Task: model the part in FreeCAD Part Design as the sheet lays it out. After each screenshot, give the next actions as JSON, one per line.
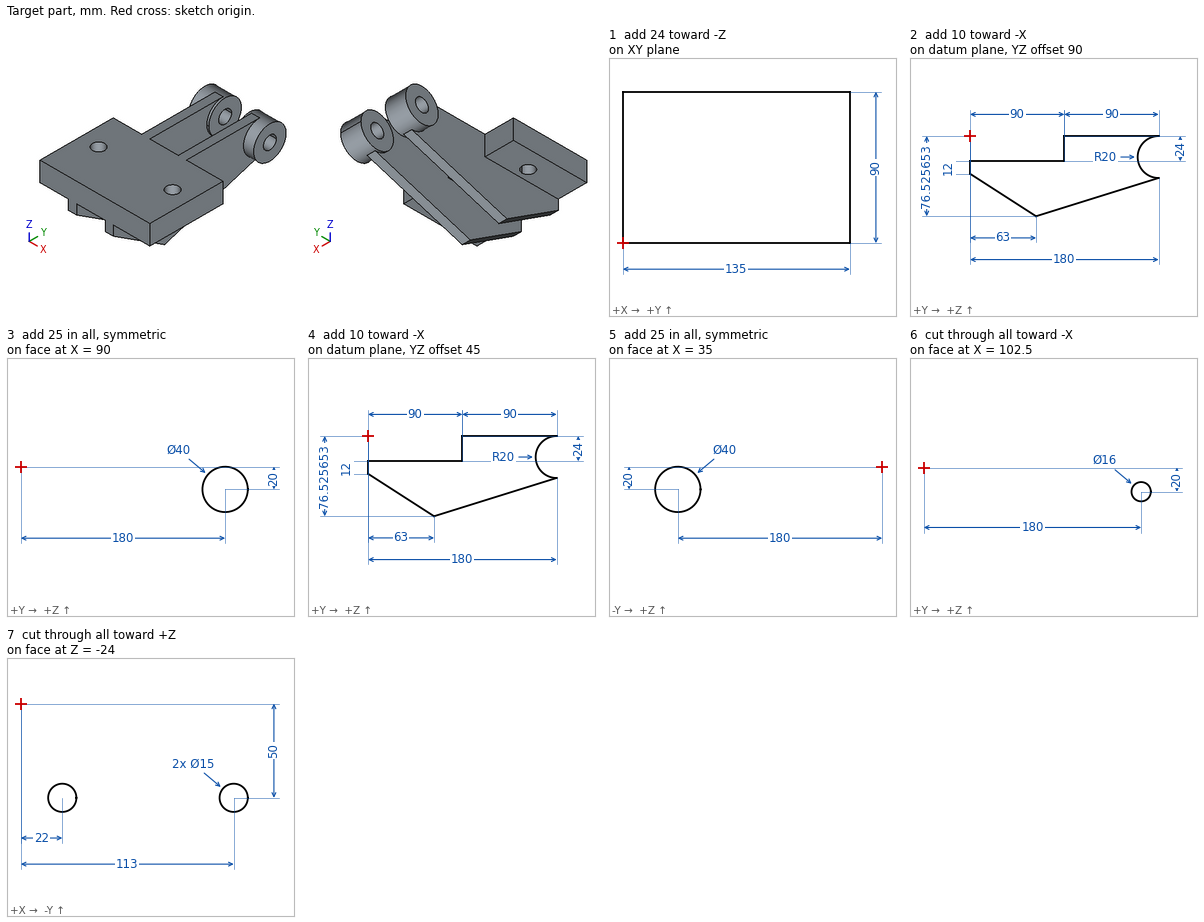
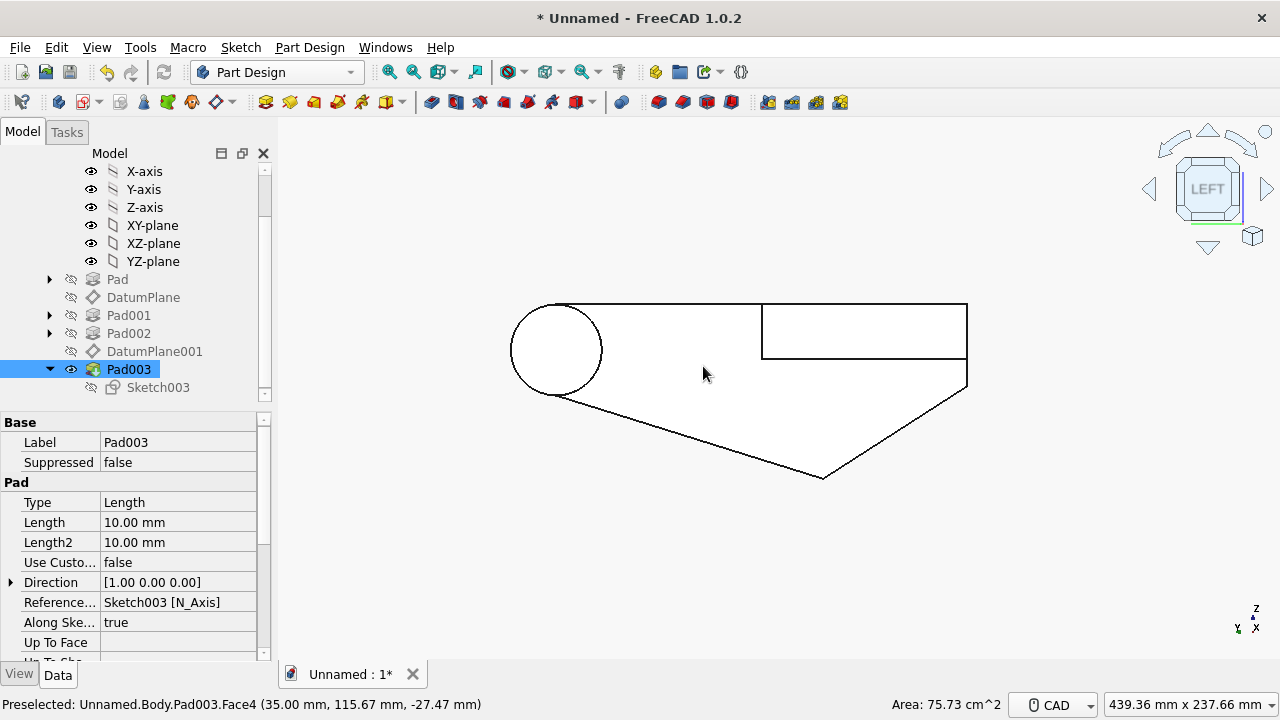
{"action": "left_click", "coordinate": [84, 102]}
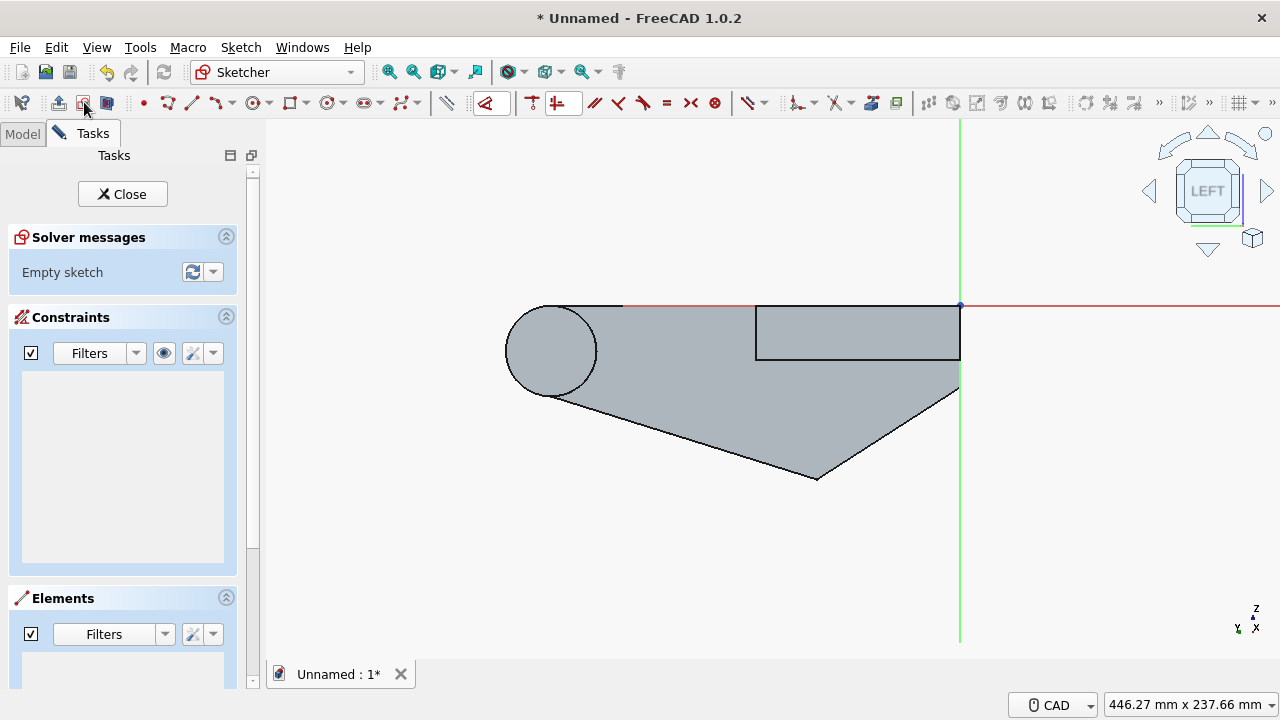
{"action": "scroll", "coordinate": [501, 339], "scroll_direction": "up", "scroll_amount": 7}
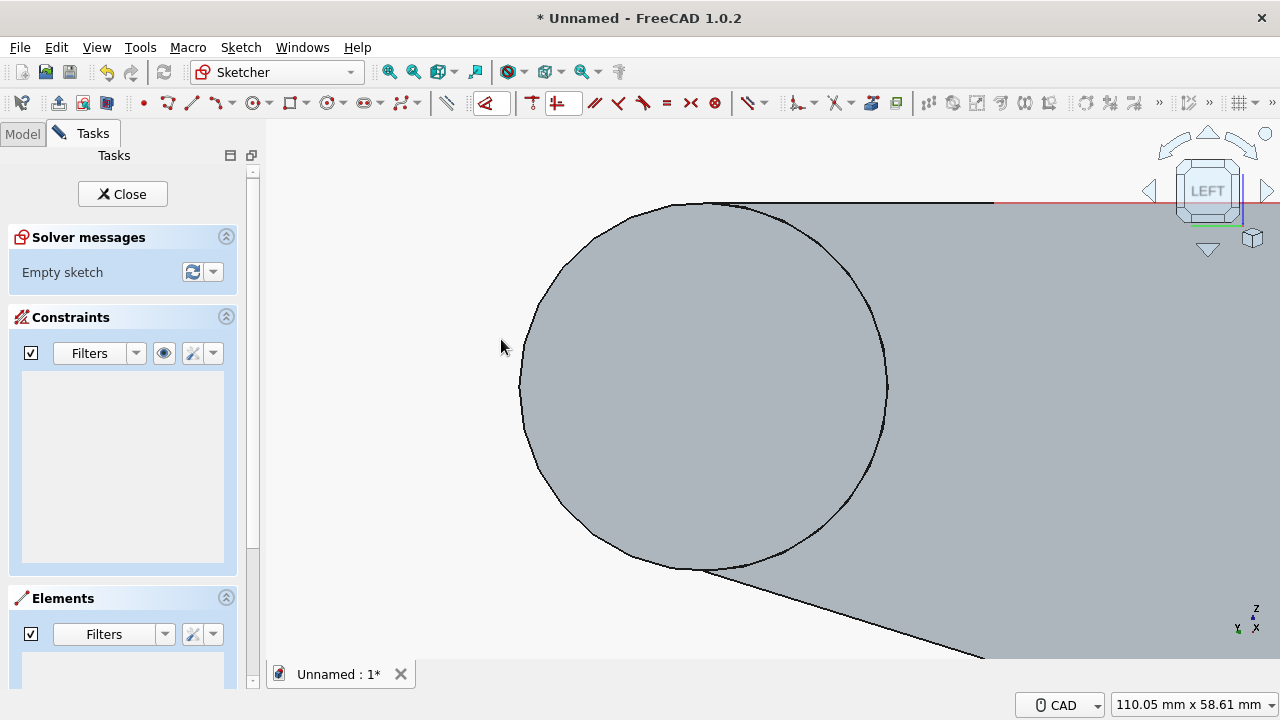
{"action": "key", "text": "g c"}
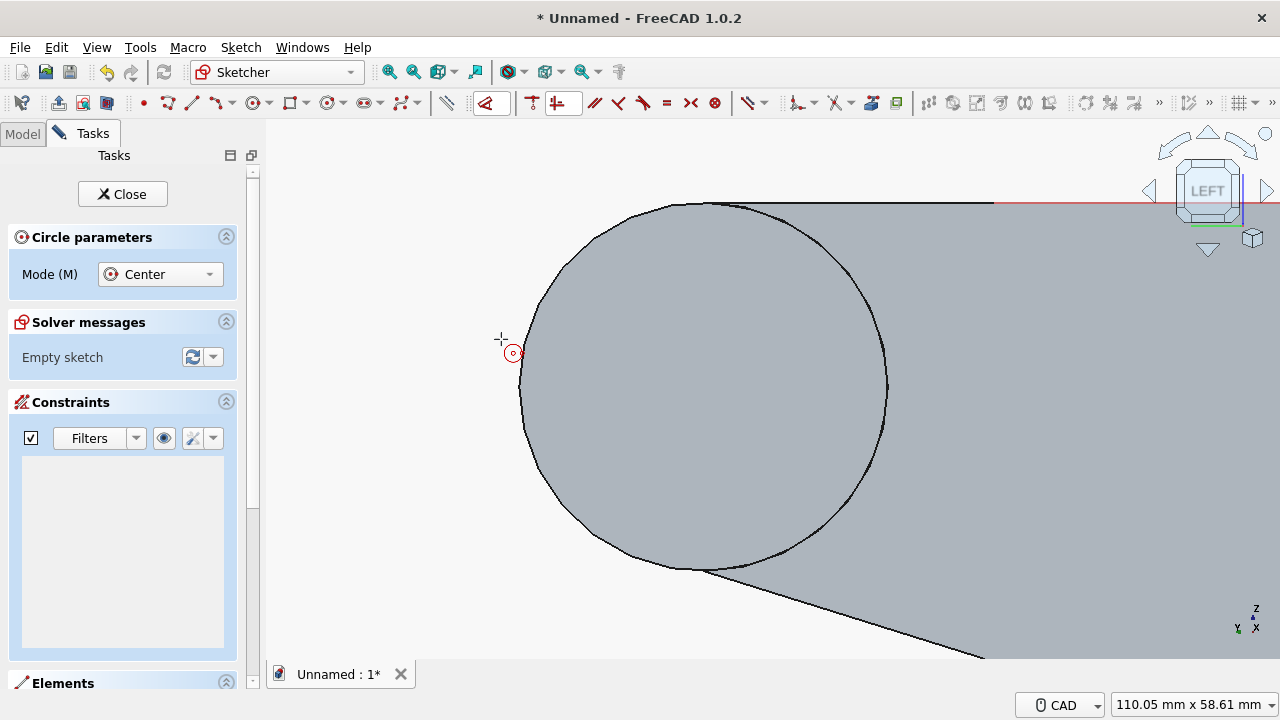
{"action": "left_click", "coordinate": [704, 387]}
{"action": "mouse_move", "coordinate": [834, 257]}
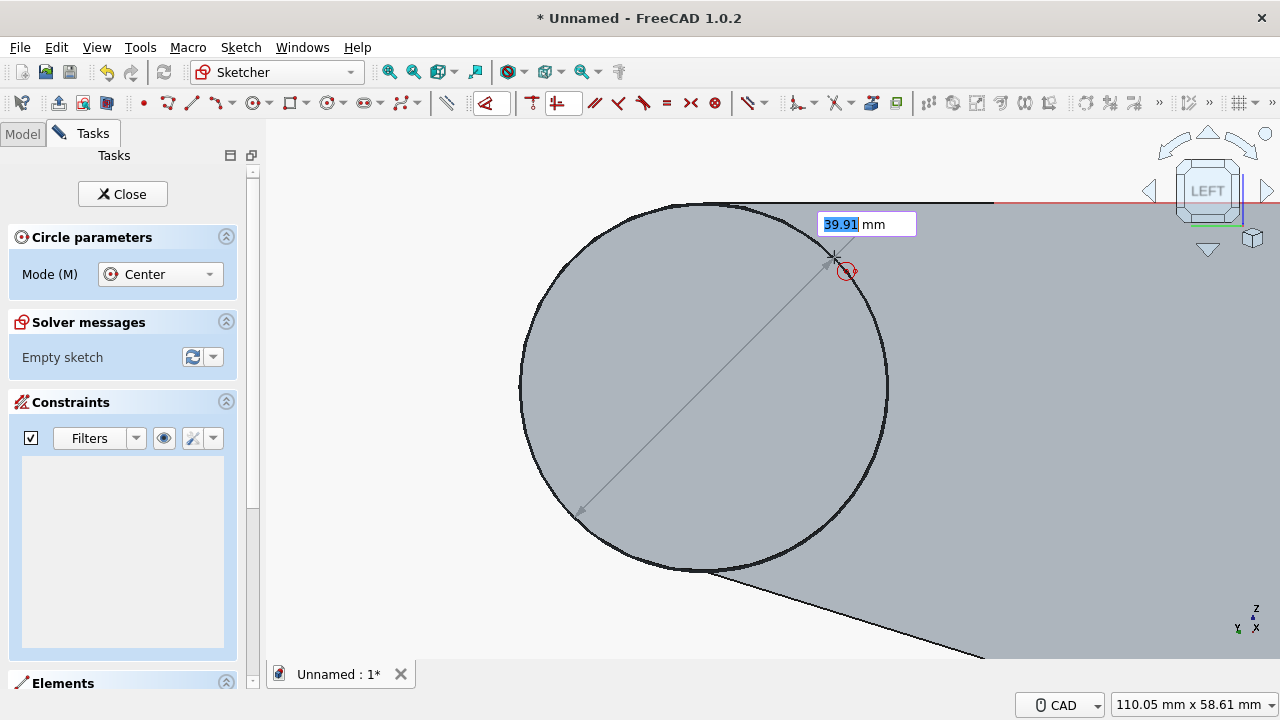
{"action": "type", "text": "40"}
{"action": "key", "text": "Return"}
{"action": "key", "text": "Escape"}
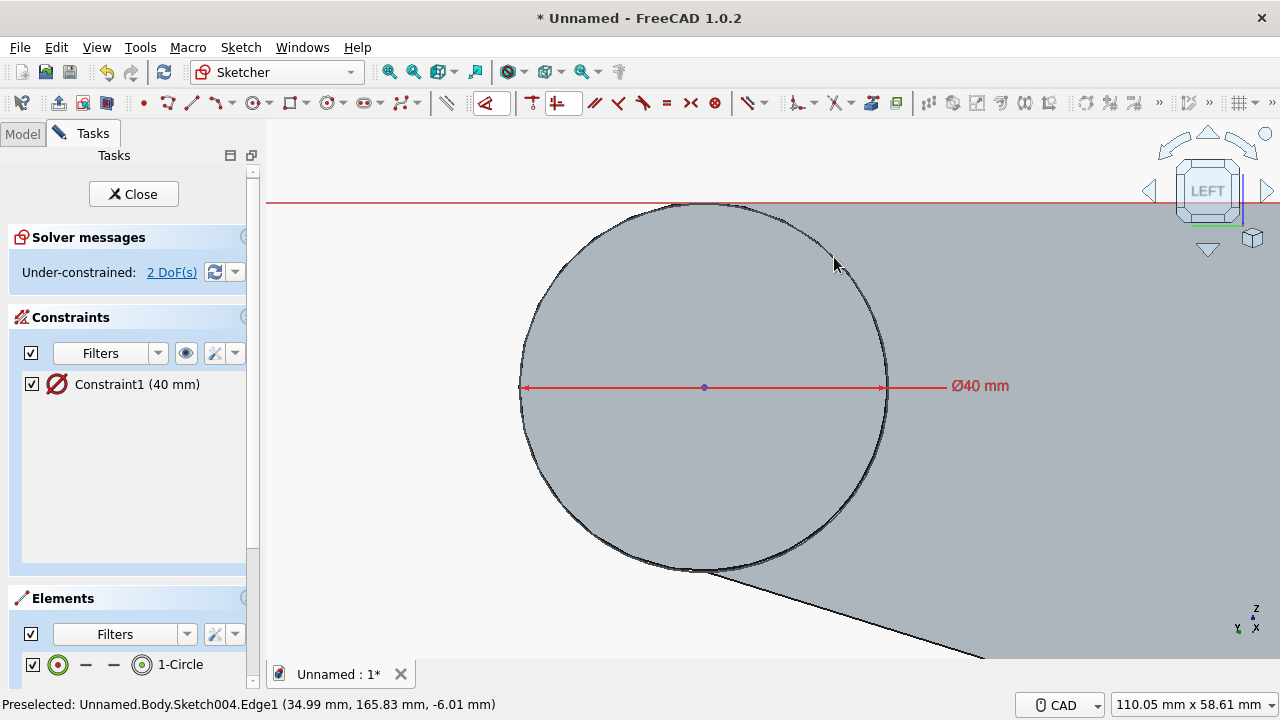
{"action": "left_click", "coordinate": [704, 388]}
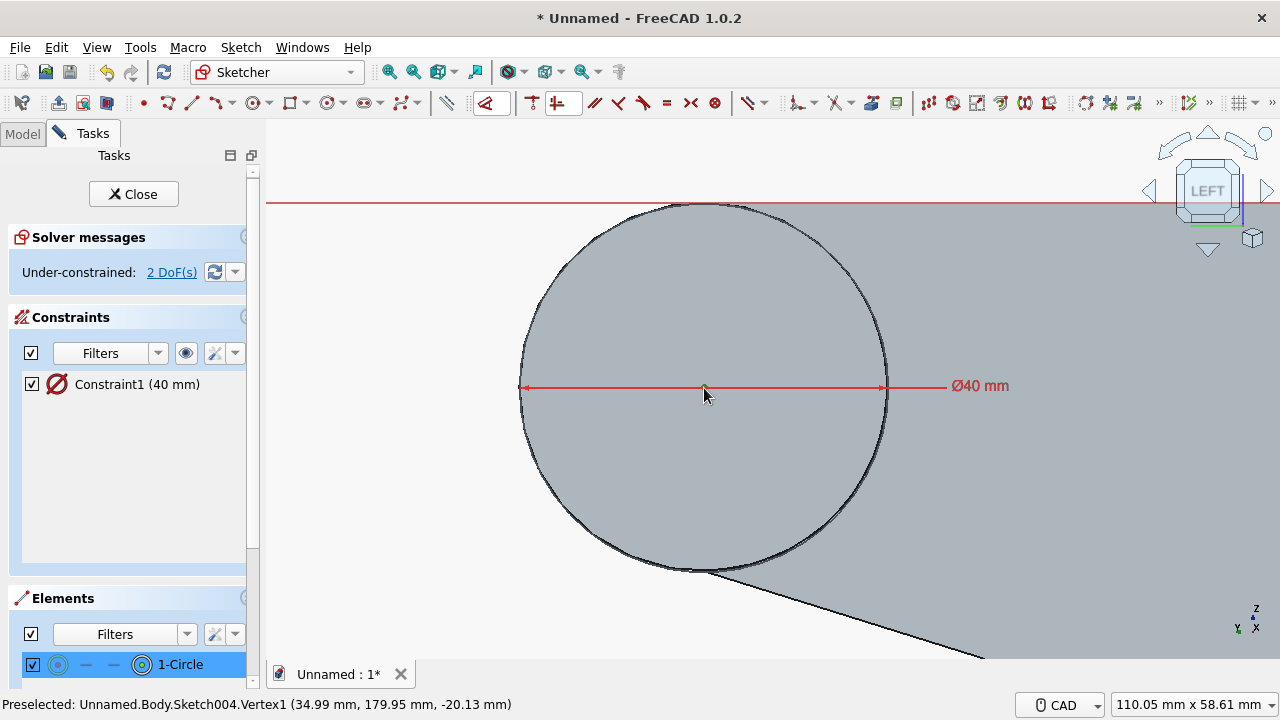
{"action": "left_click", "coordinate": [504, 104]}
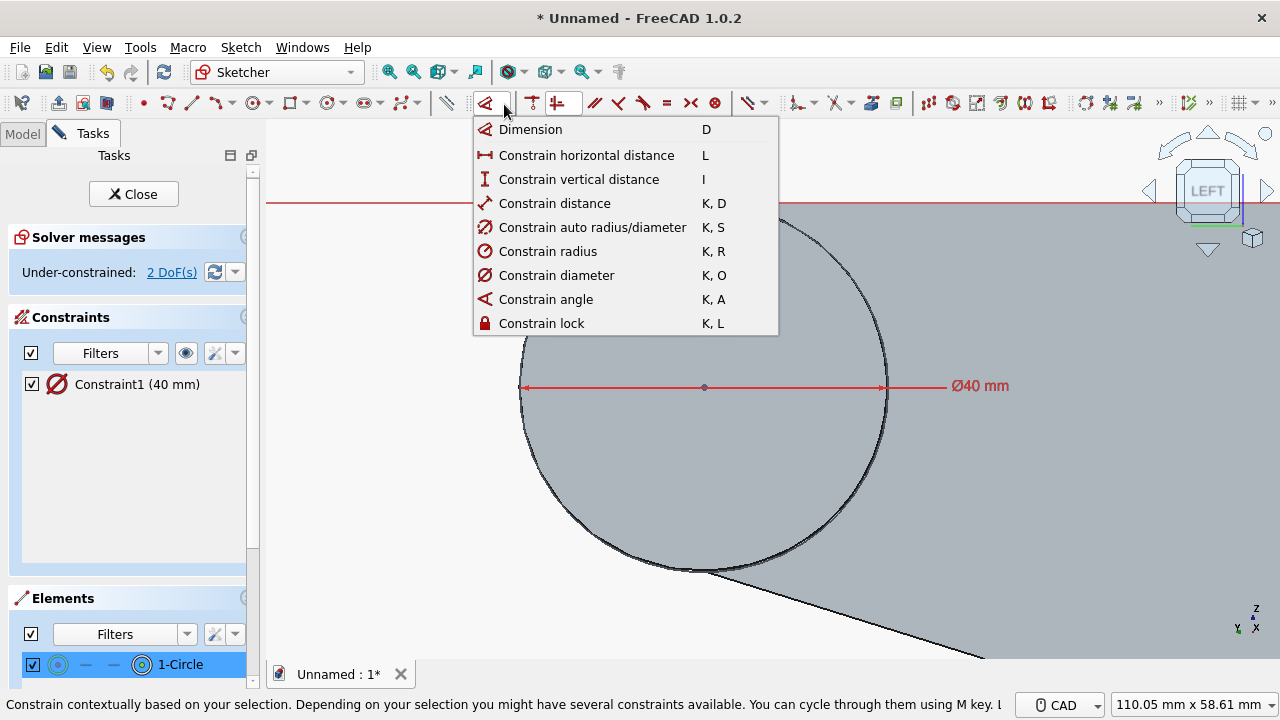
{"action": "left_click", "coordinate": [626, 179]}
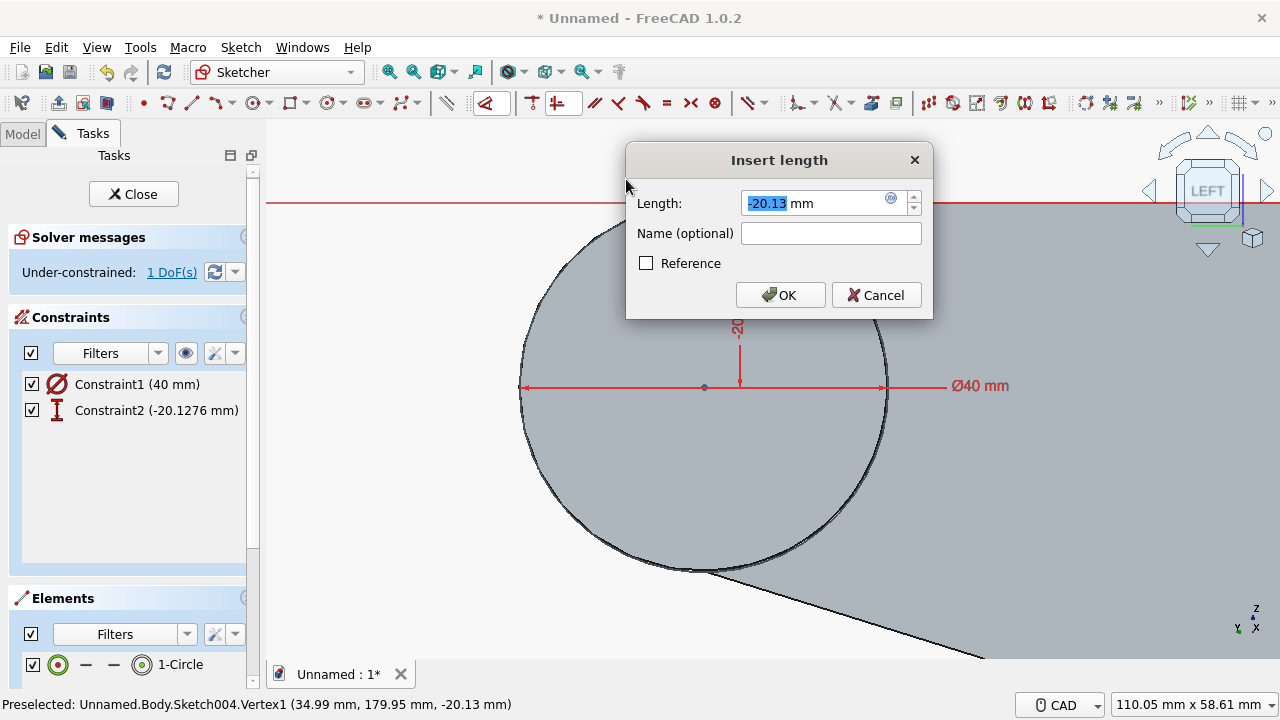
{"action": "type", "text": "-20"}
{"action": "key", "text": "Return"}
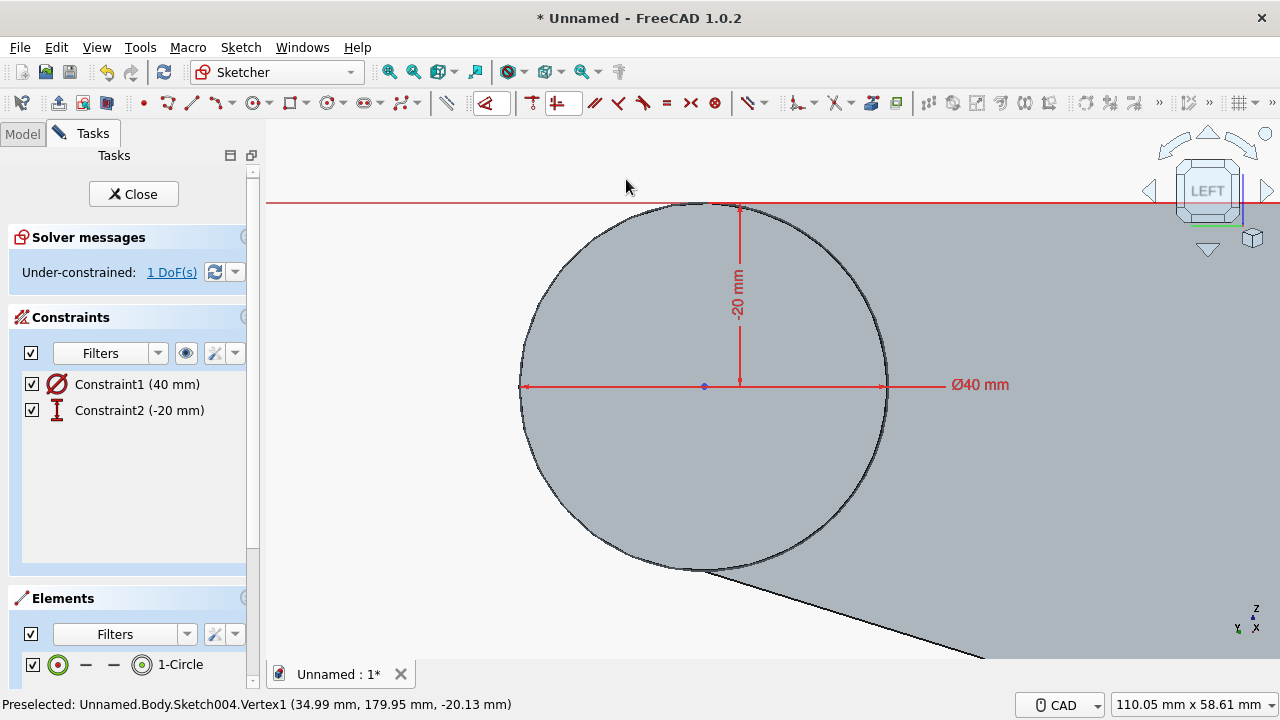
{"action": "left_click", "coordinate": [704, 387]}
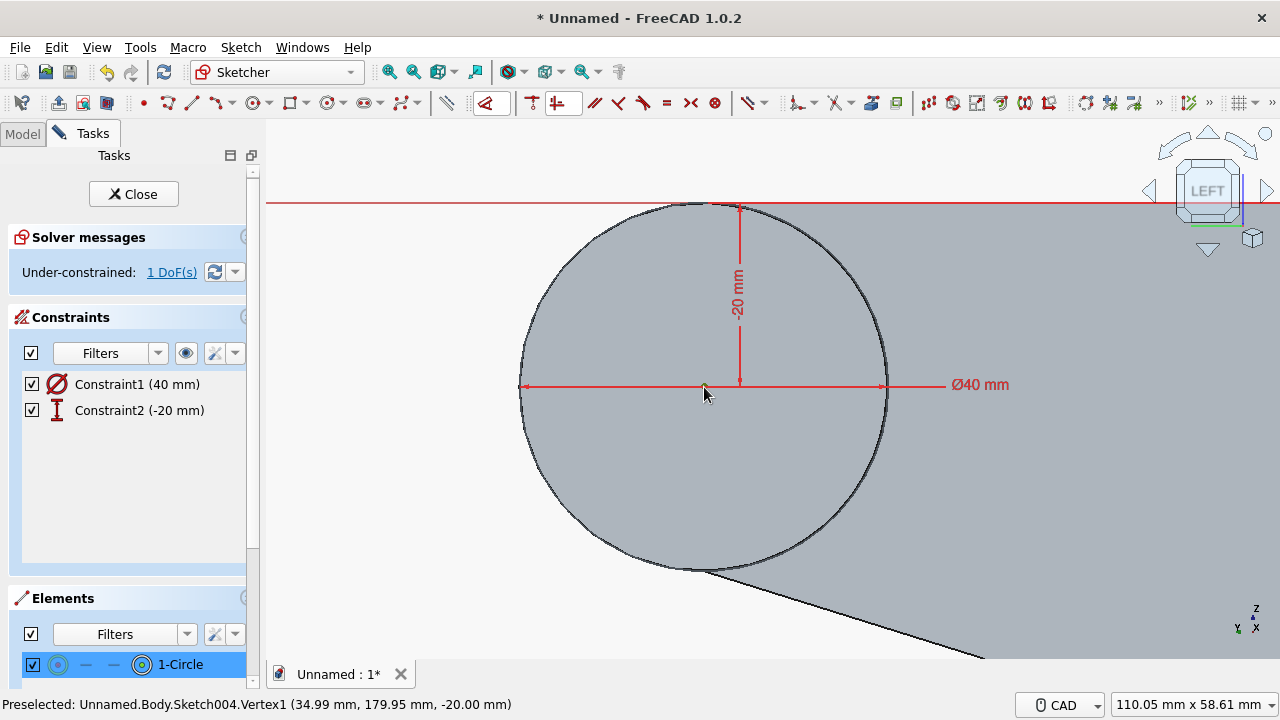
{"action": "key", "text": "l"}